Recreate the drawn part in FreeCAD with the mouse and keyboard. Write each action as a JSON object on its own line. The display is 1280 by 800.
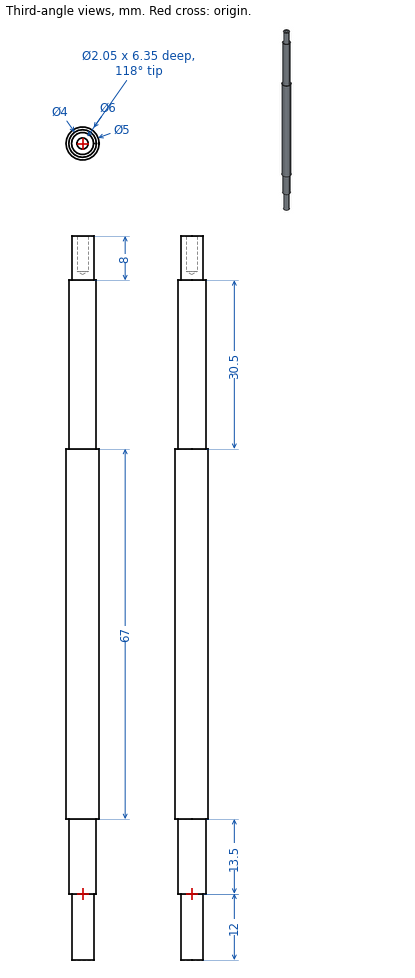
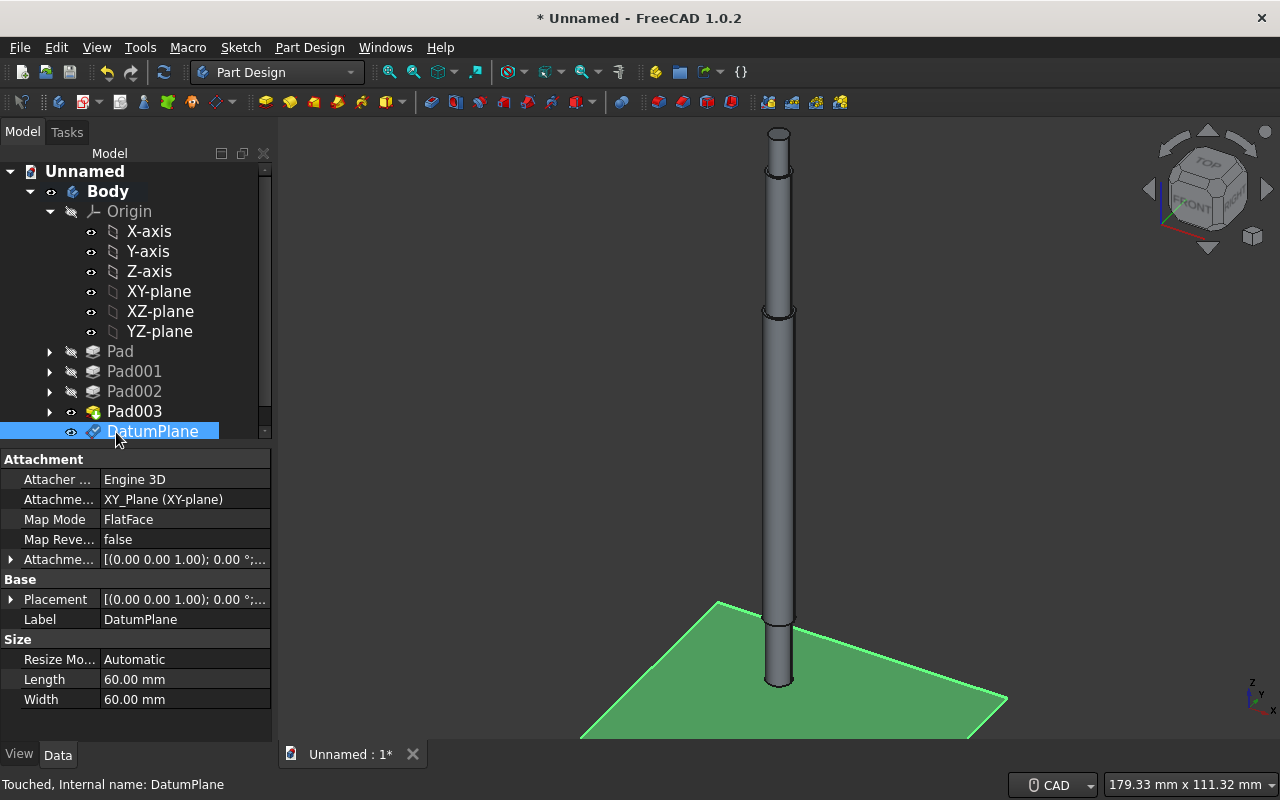
{"action": "left_click", "coordinate": [84, 102]}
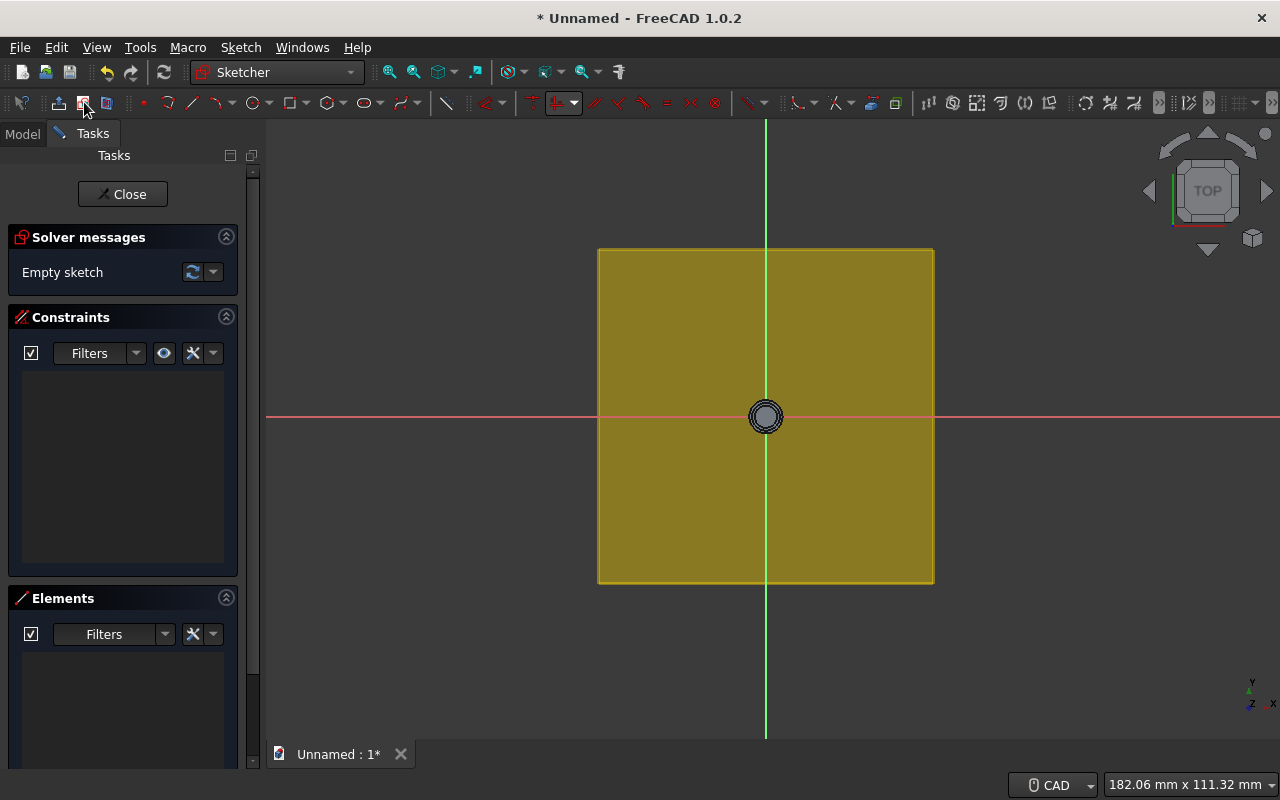
{"action": "left_click", "coordinate": [108, 104]}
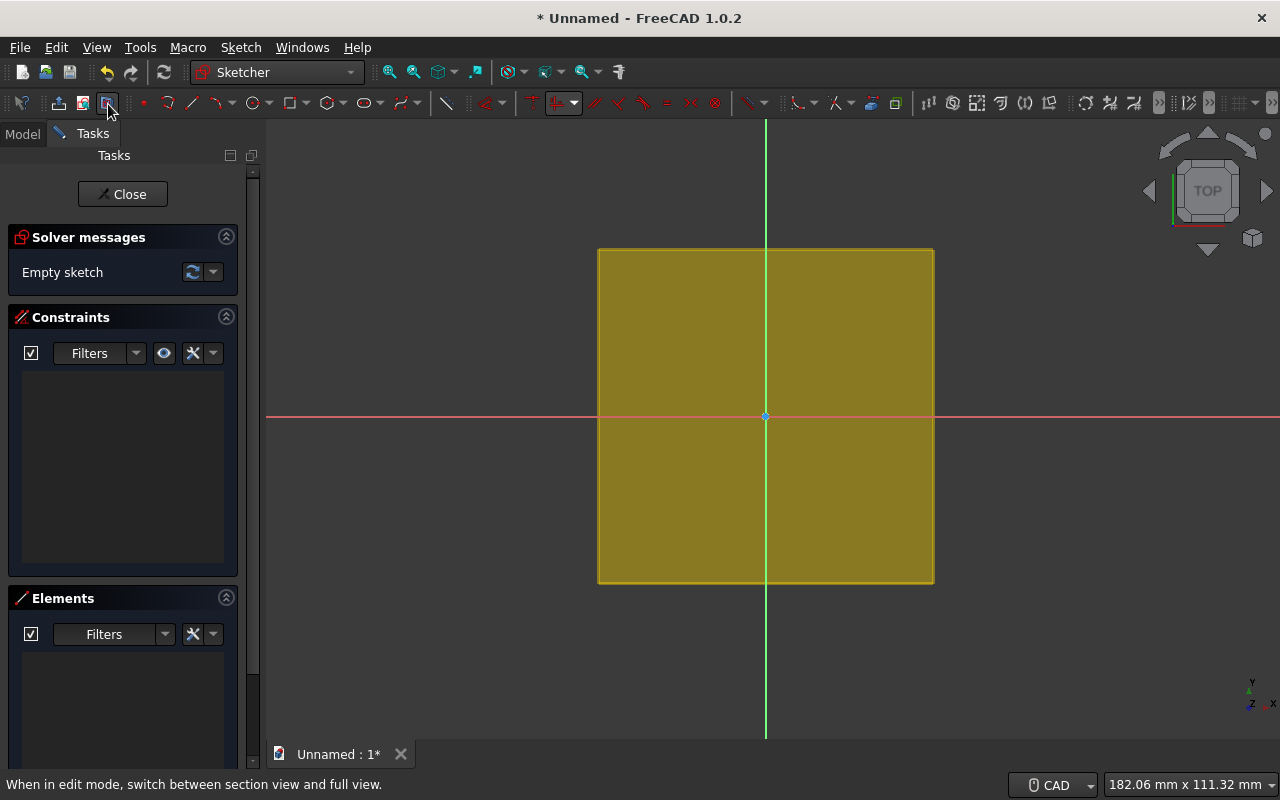
{"action": "scroll", "coordinate": [770, 416], "scroll_direction": "up", "scroll_amount": 14}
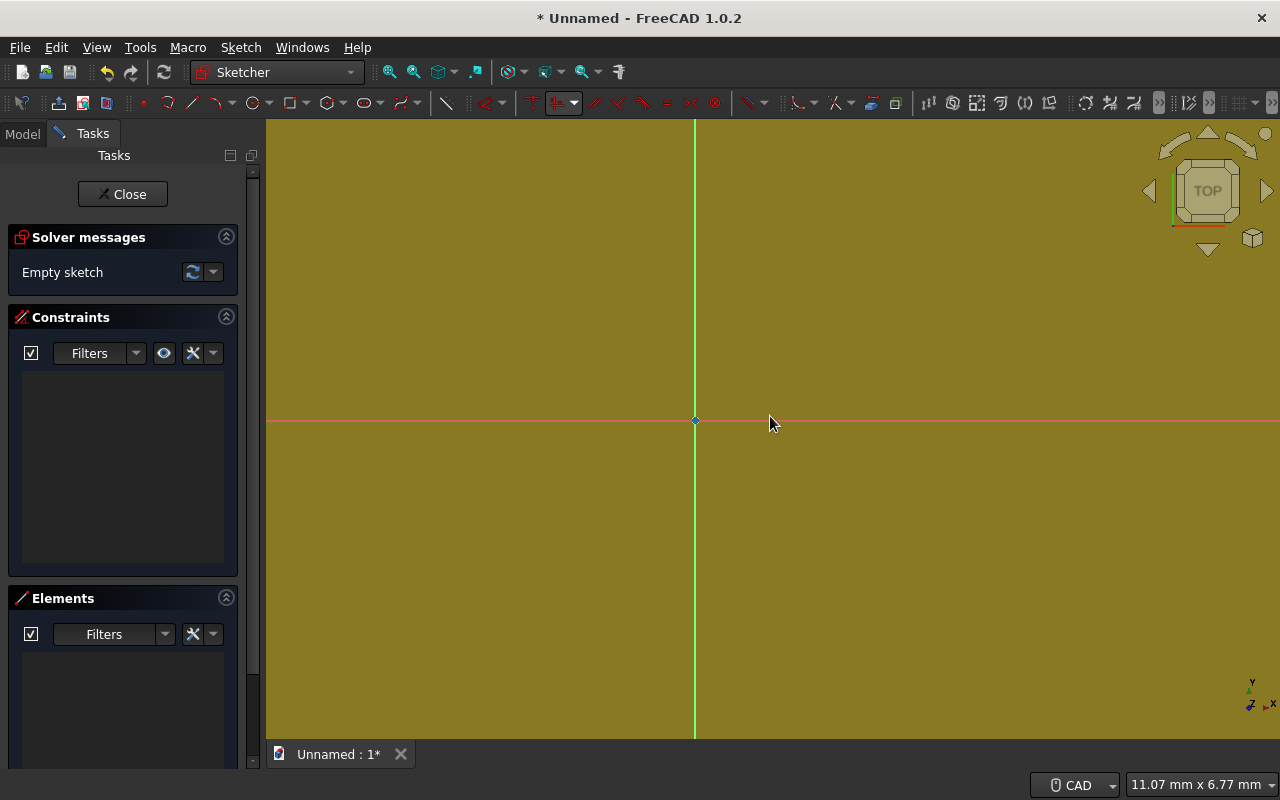
{"action": "left_click", "coordinate": [254, 104]}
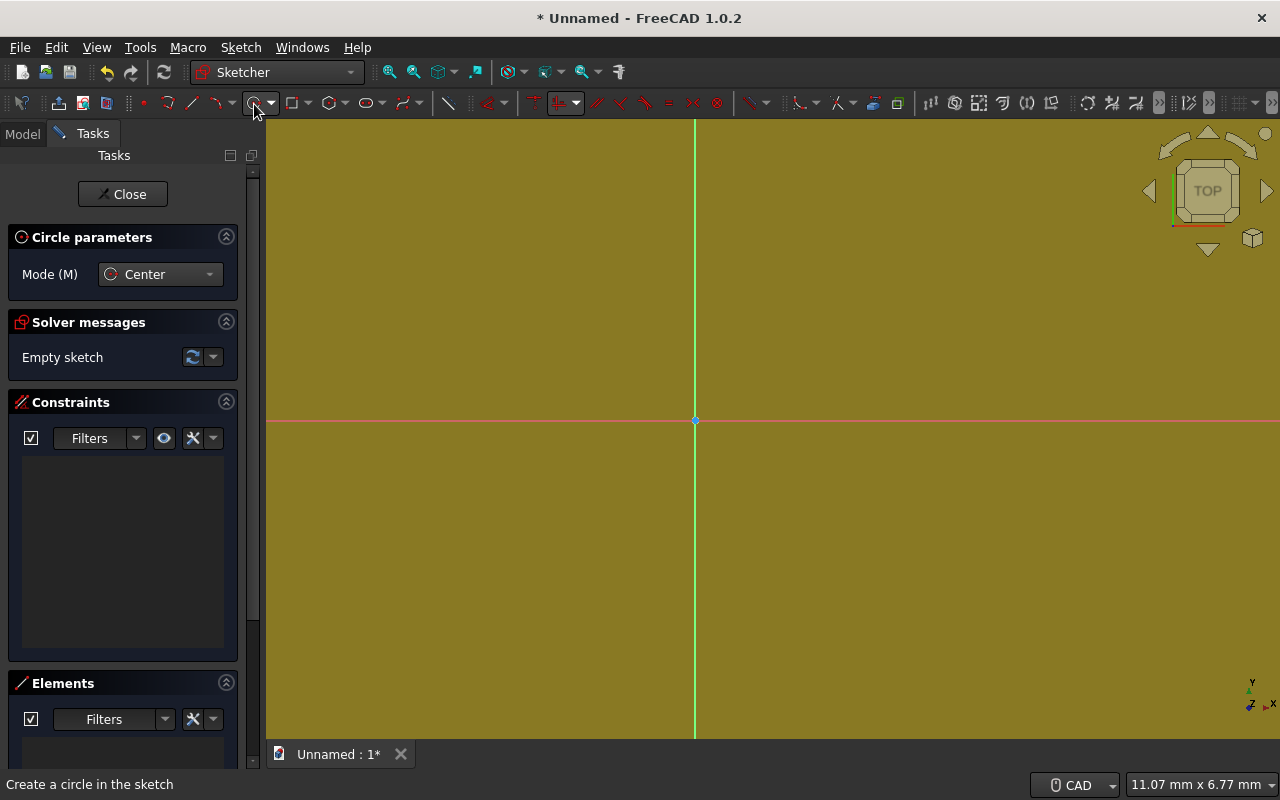
{"action": "left_click", "coordinate": [695, 421]}
{"action": "left_click", "coordinate": [825, 291]}
{"action": "key", "text": "Escape"}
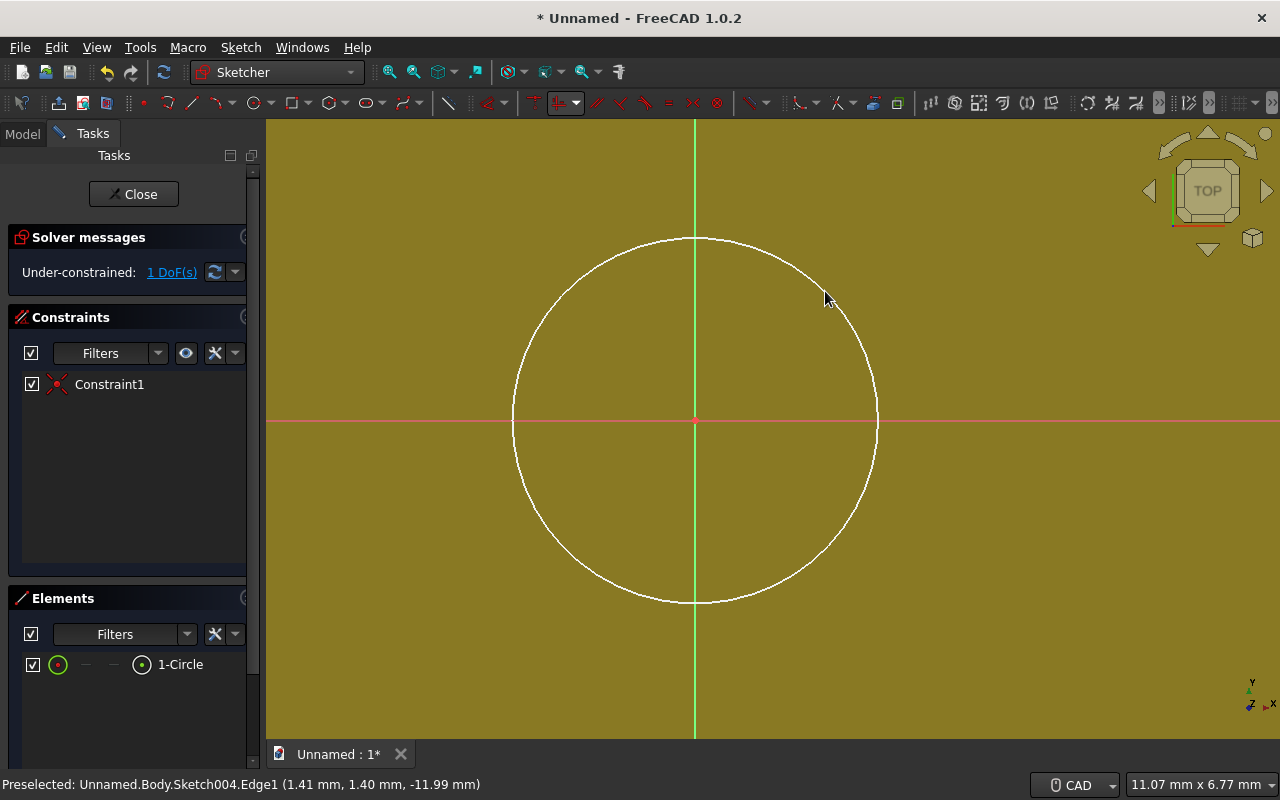
{"action": "left_click", "coordinate": [488, 104]}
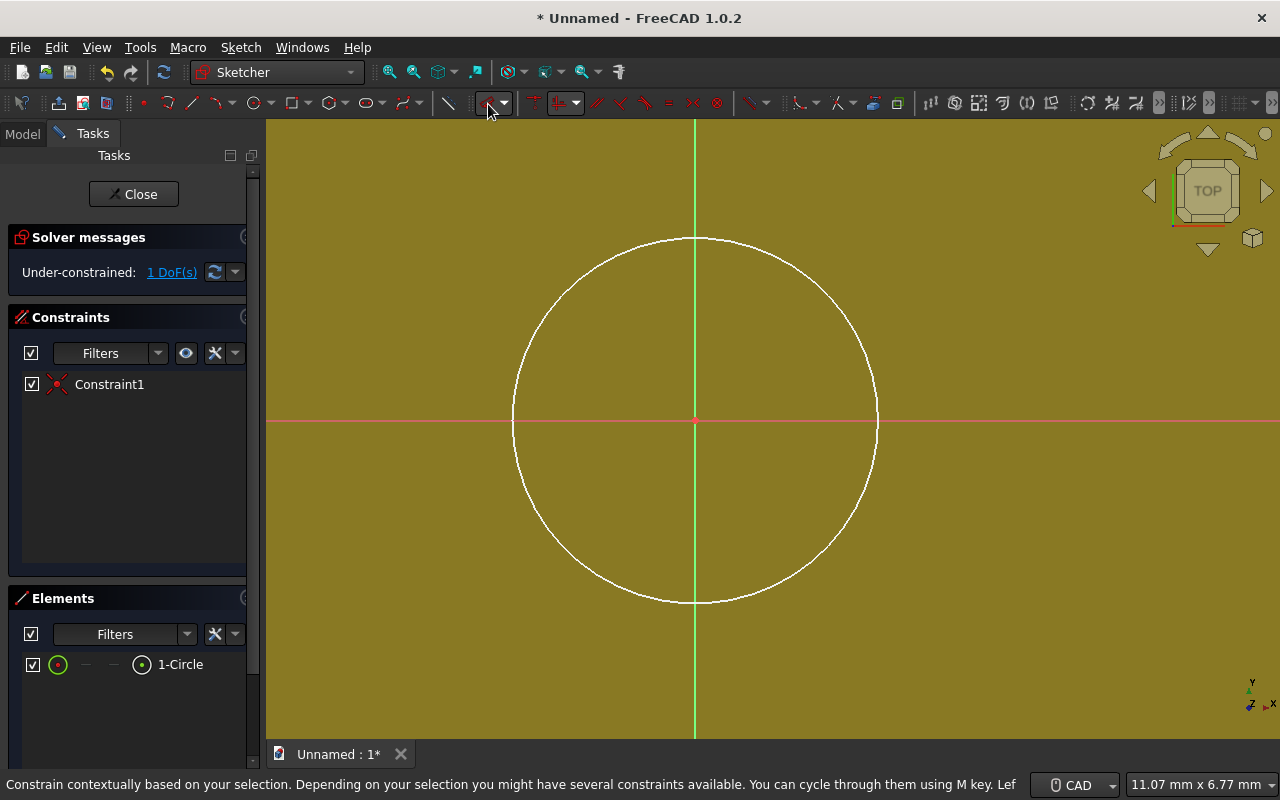
{"action": "left_click", "coordinate": [824, 291]}
{"action": "left_click", "coordinate": [847, 268]}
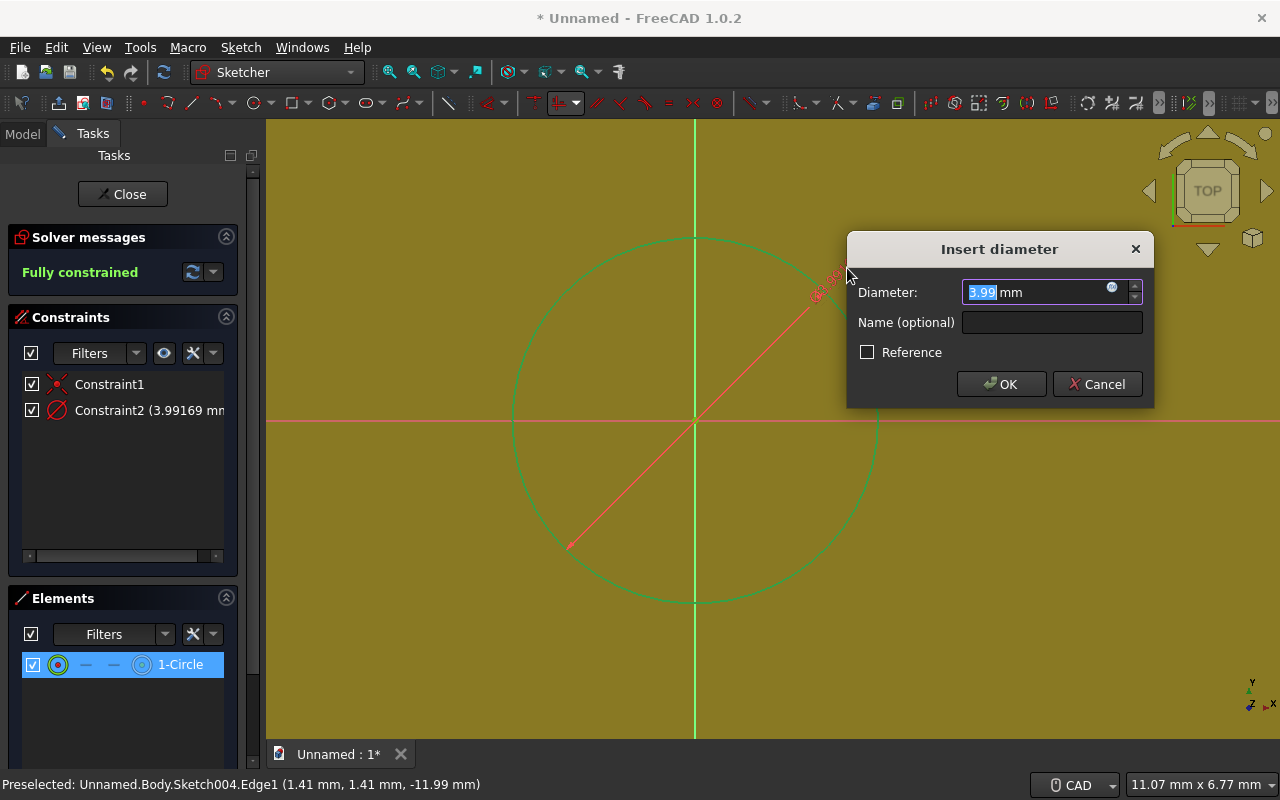
{"action": "type", "text": "4"}
{"action": "key", "text": "Return"}
{"action": "key", "text": "Escape"}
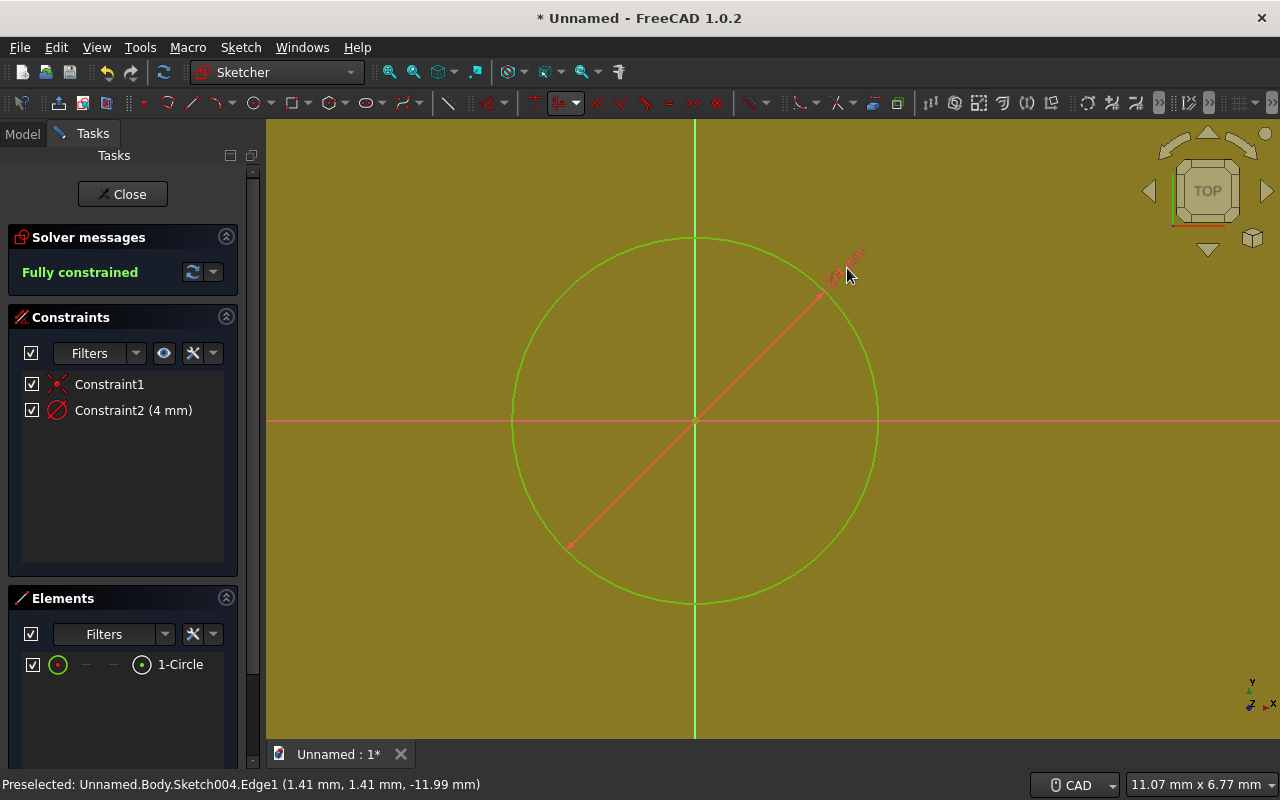
{"action": "left_click", "coordinate": [123, 194]}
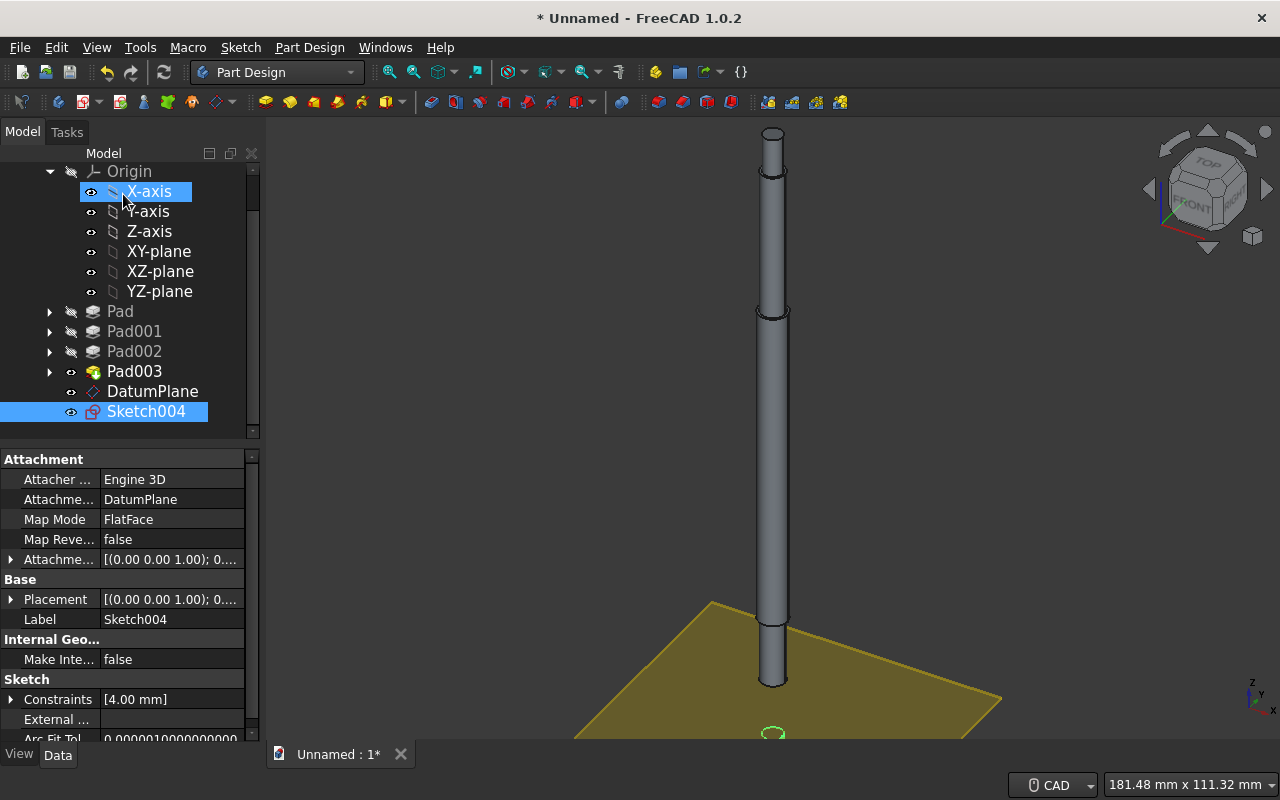
{"action": "left_click", "coordinate": [266, 102]}